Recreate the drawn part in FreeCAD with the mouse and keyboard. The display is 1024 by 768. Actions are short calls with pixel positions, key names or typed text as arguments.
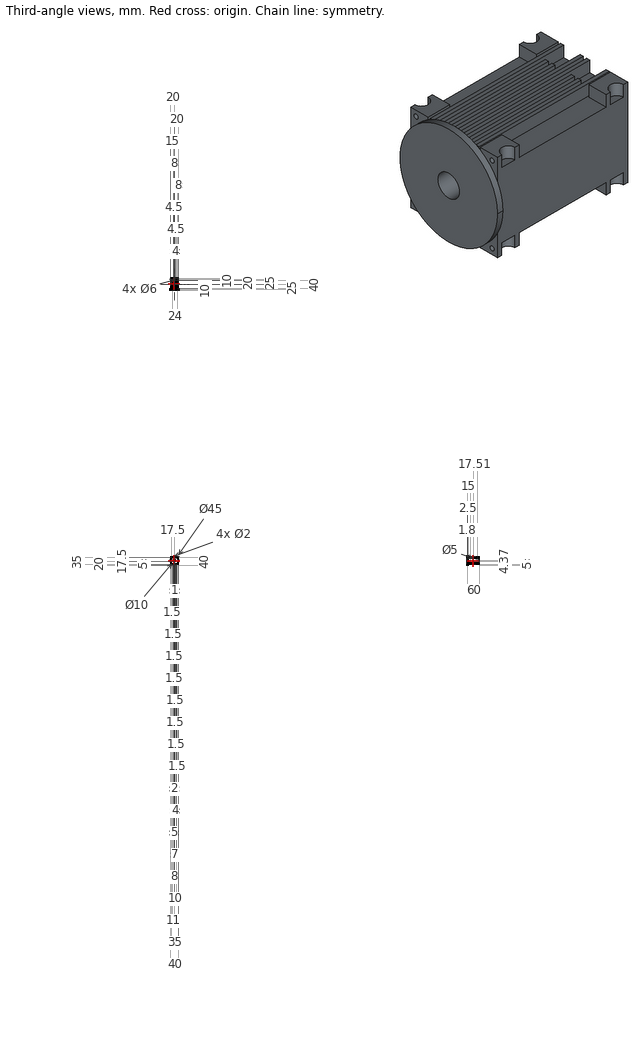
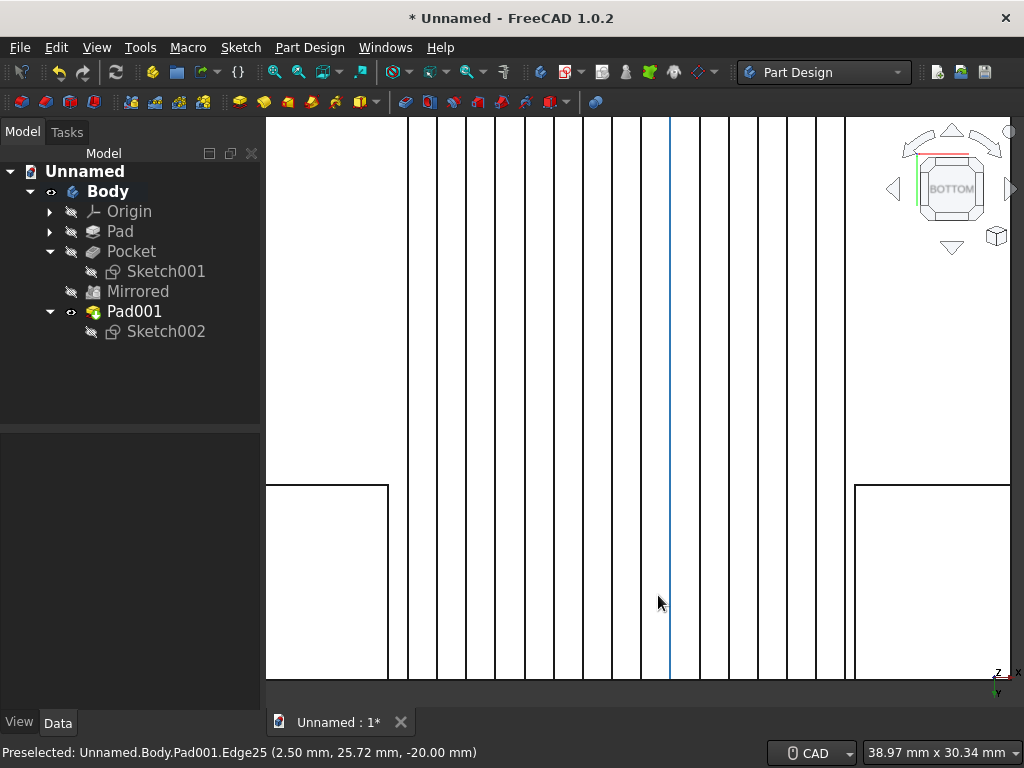
click(656, 595)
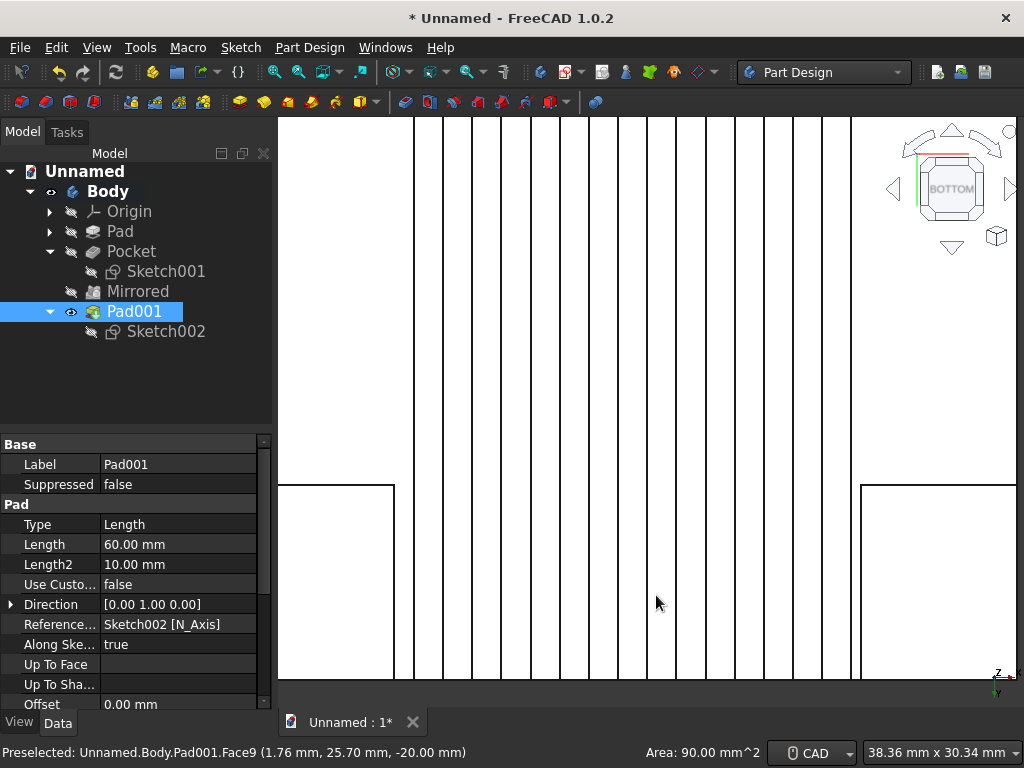
click(566, 72)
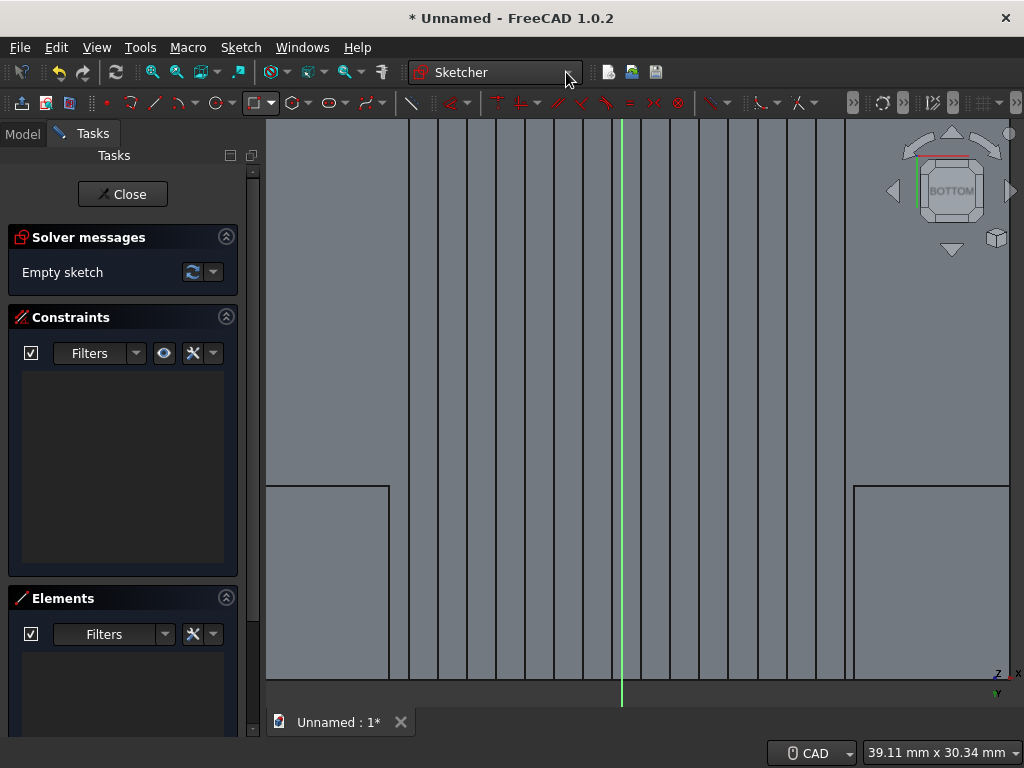
scroll(474, 462, down, 2)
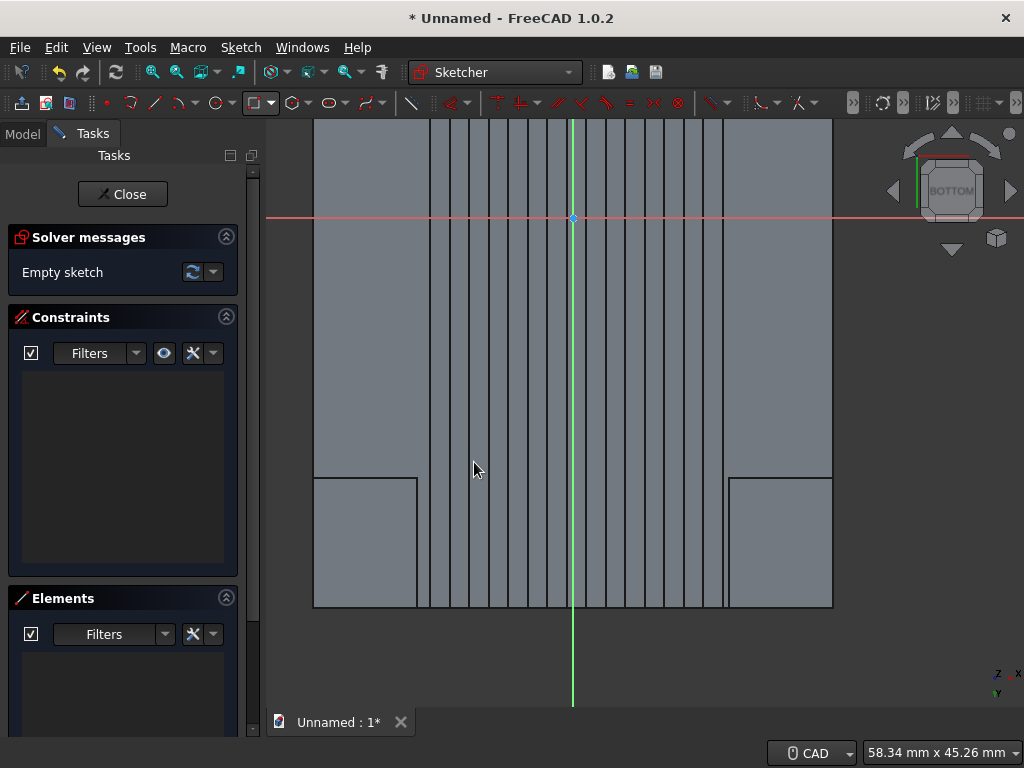
click(254, 104)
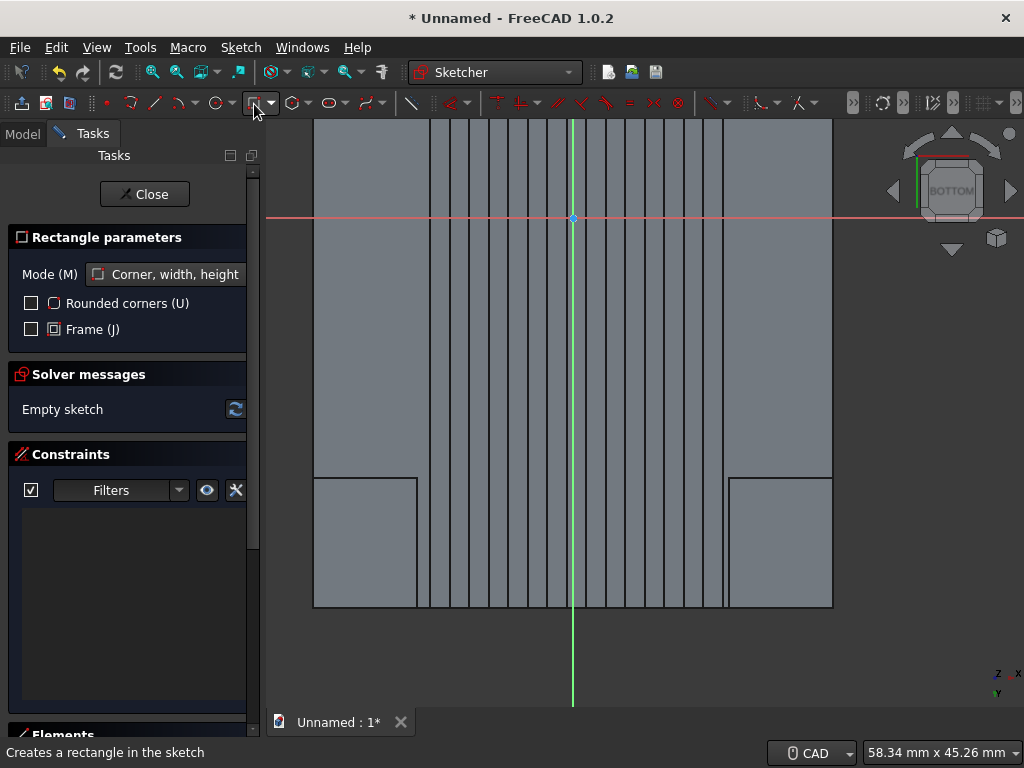
click(625, 478)
click(684, 608)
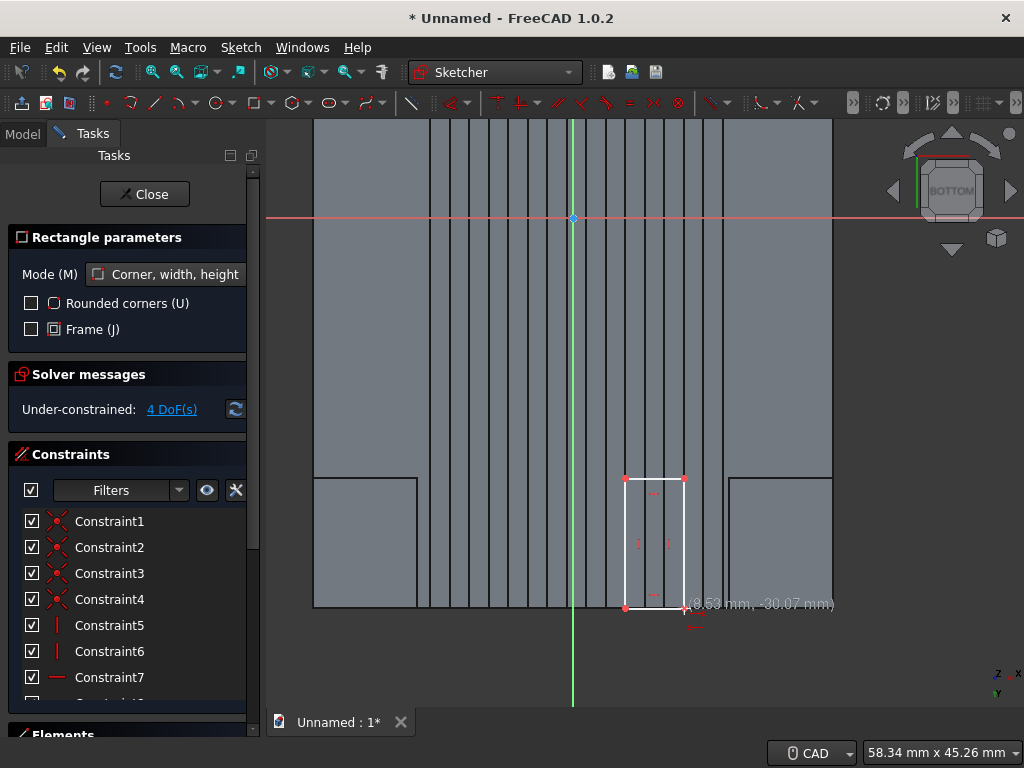
click(469, 478)
click(528, 608)
key(Escape)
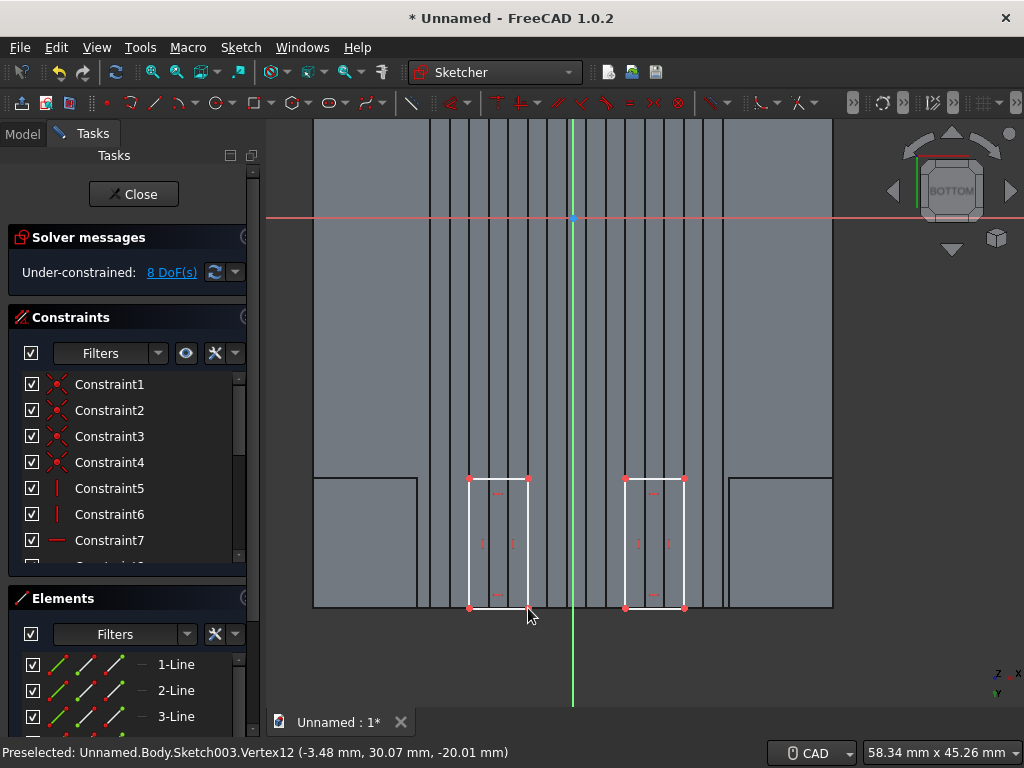
key(d)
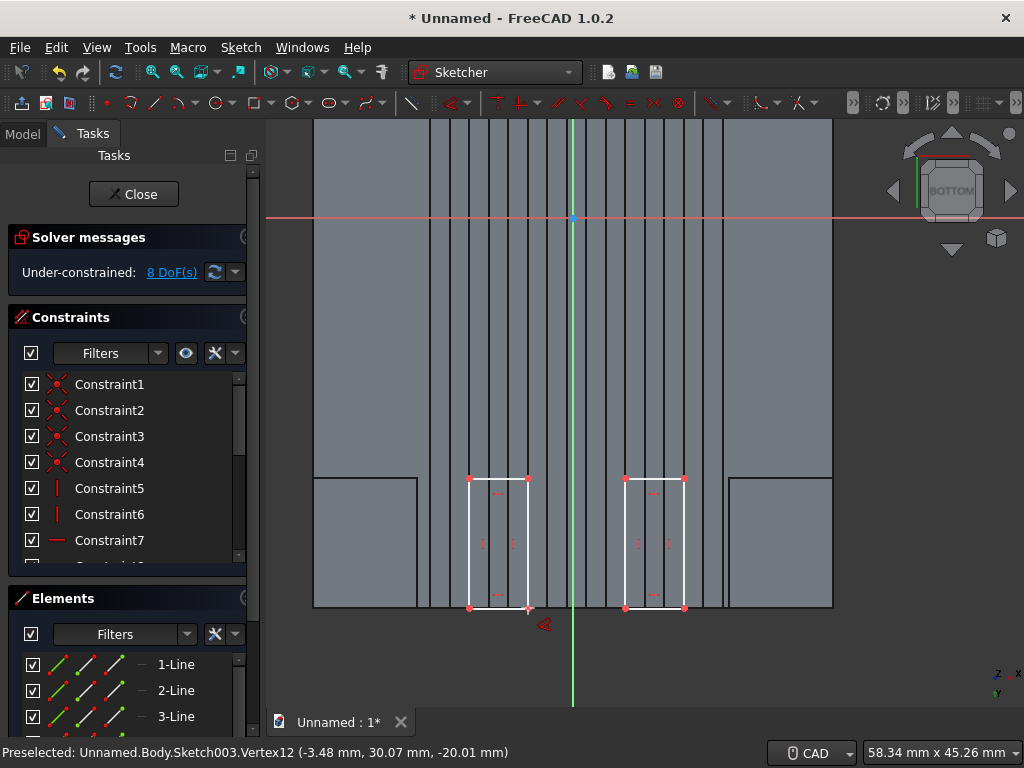
click(625, 518)
click(659, 544)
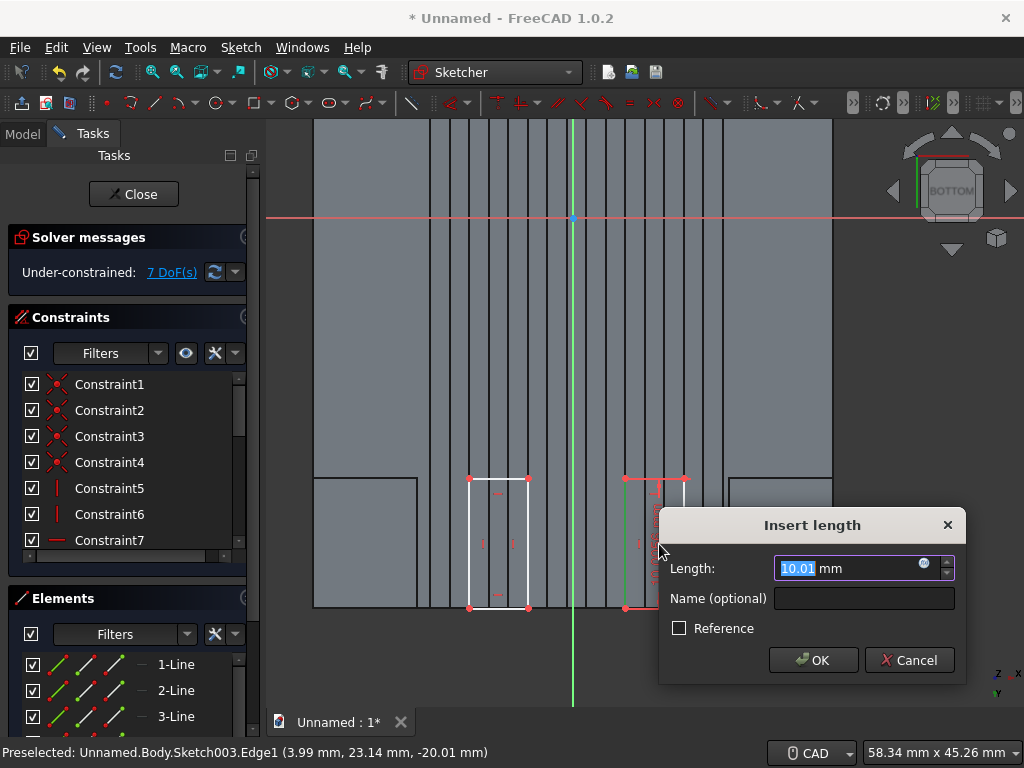
text(10)
key(Return)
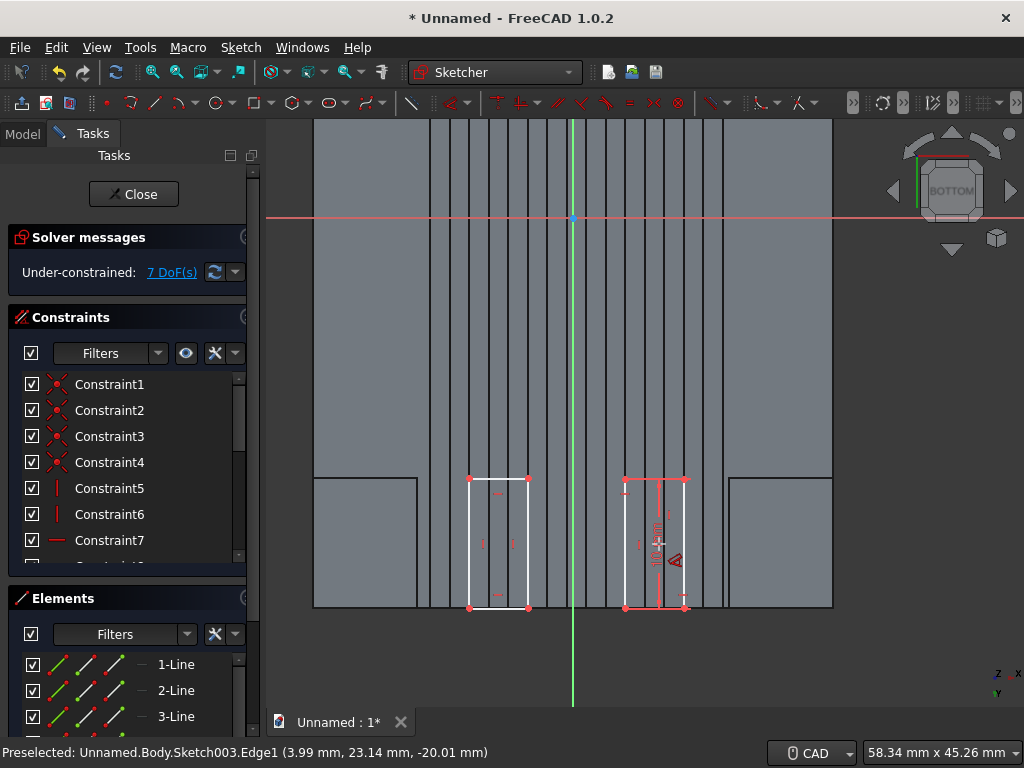
click(469, 518)
click(435, 544)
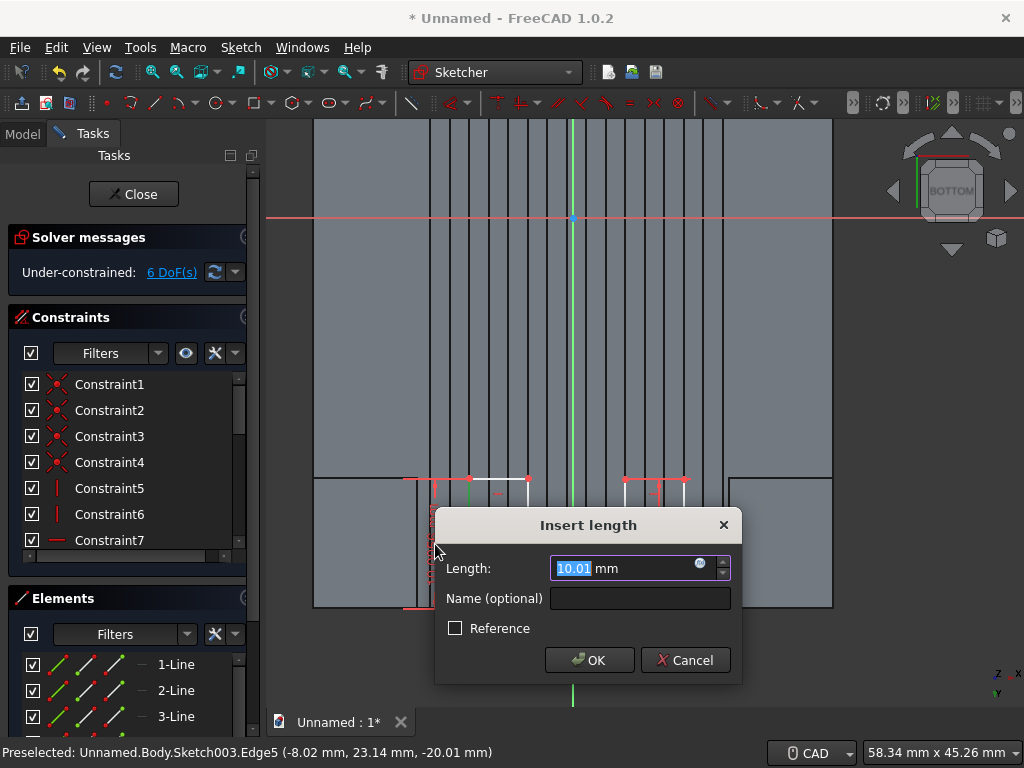
text(10)
key(Return)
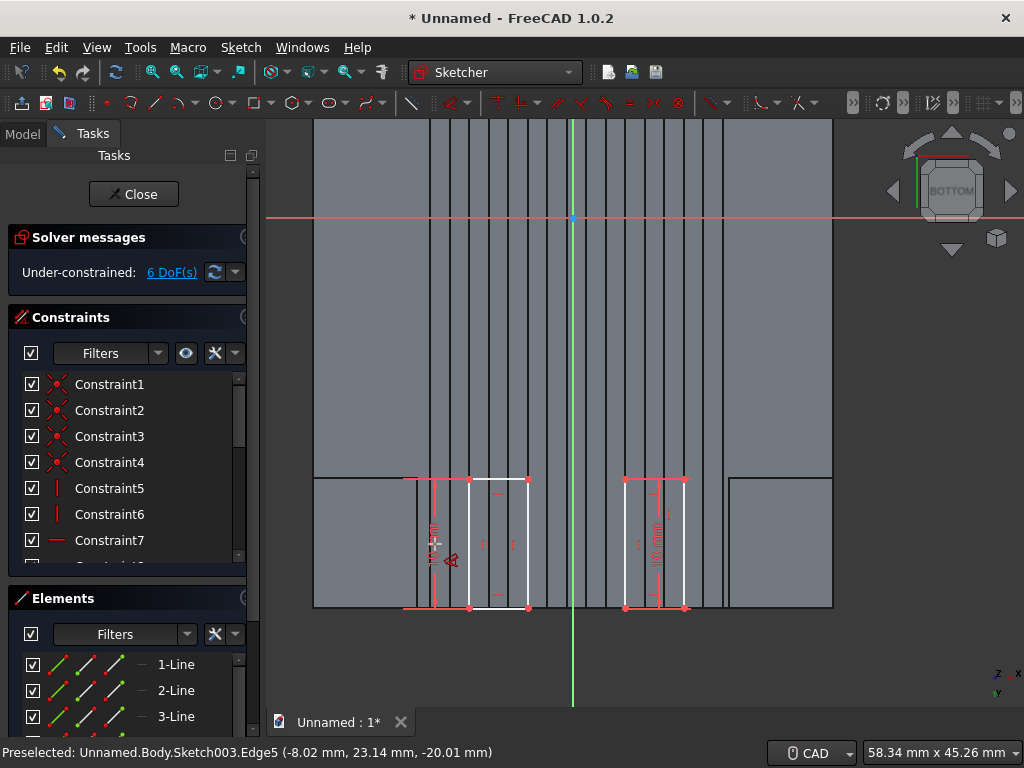
click(625, 479)
click(599, 184)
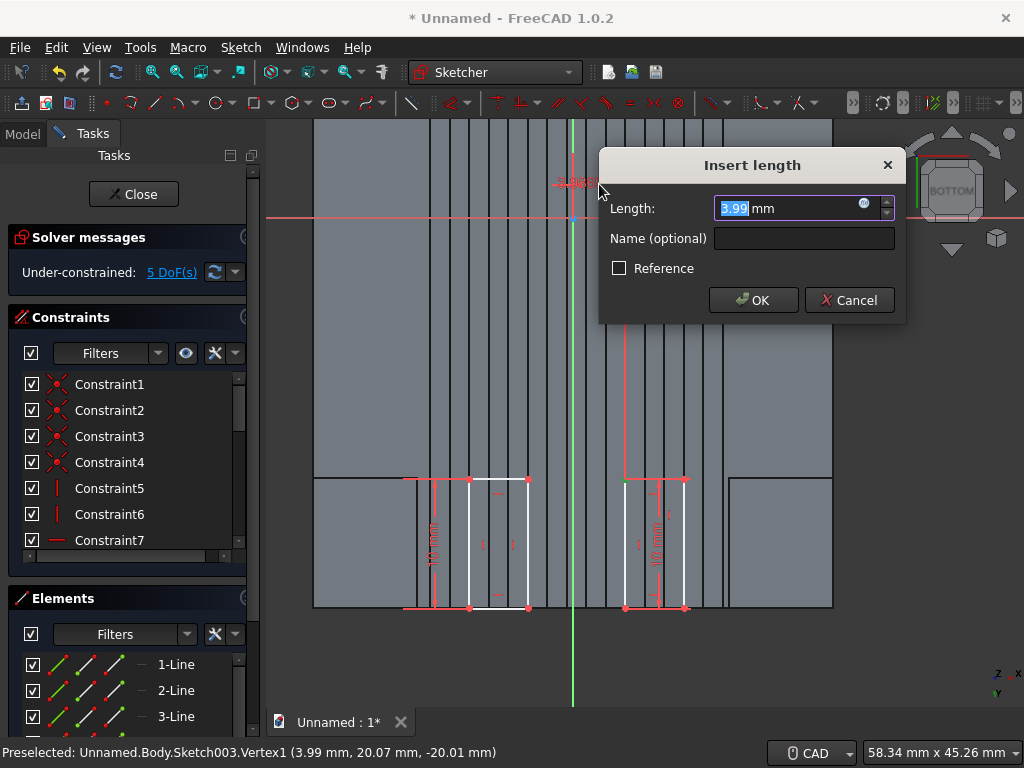
text(4)
key(Return)